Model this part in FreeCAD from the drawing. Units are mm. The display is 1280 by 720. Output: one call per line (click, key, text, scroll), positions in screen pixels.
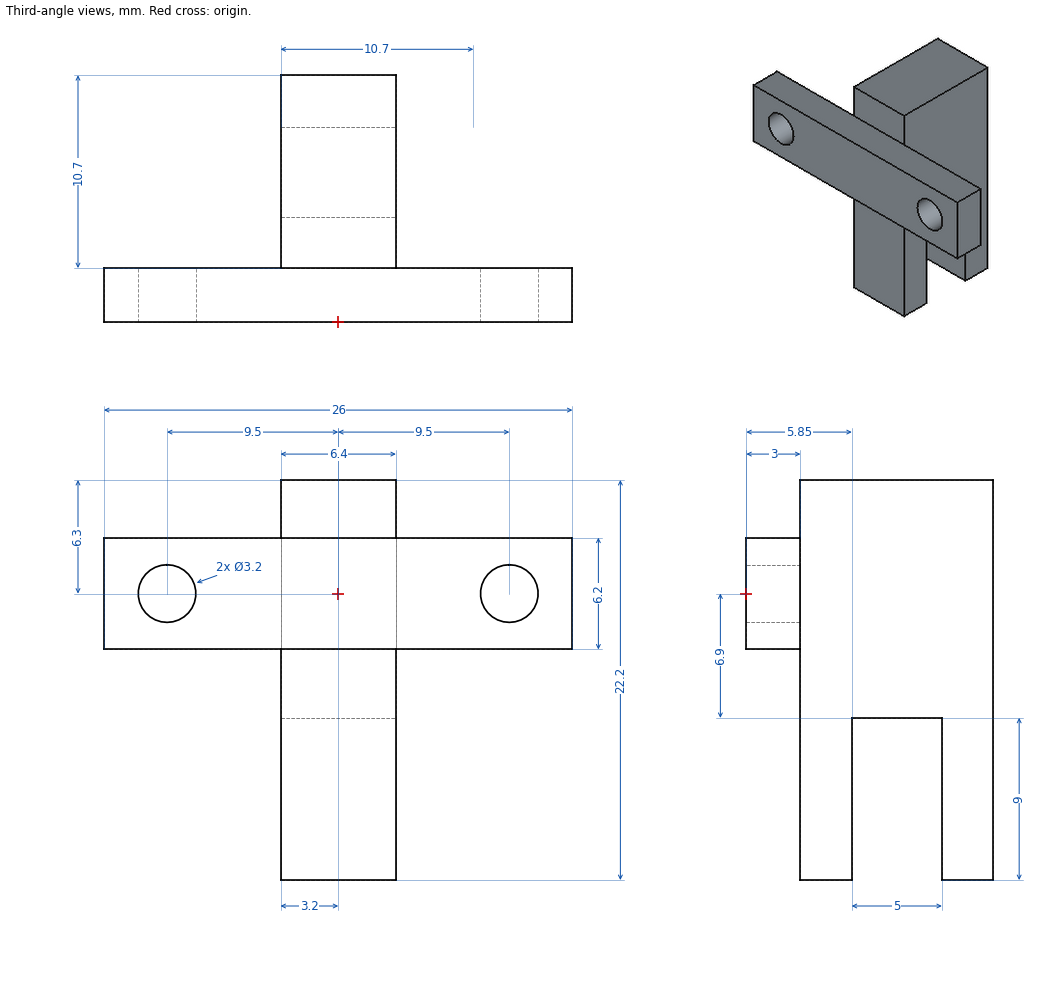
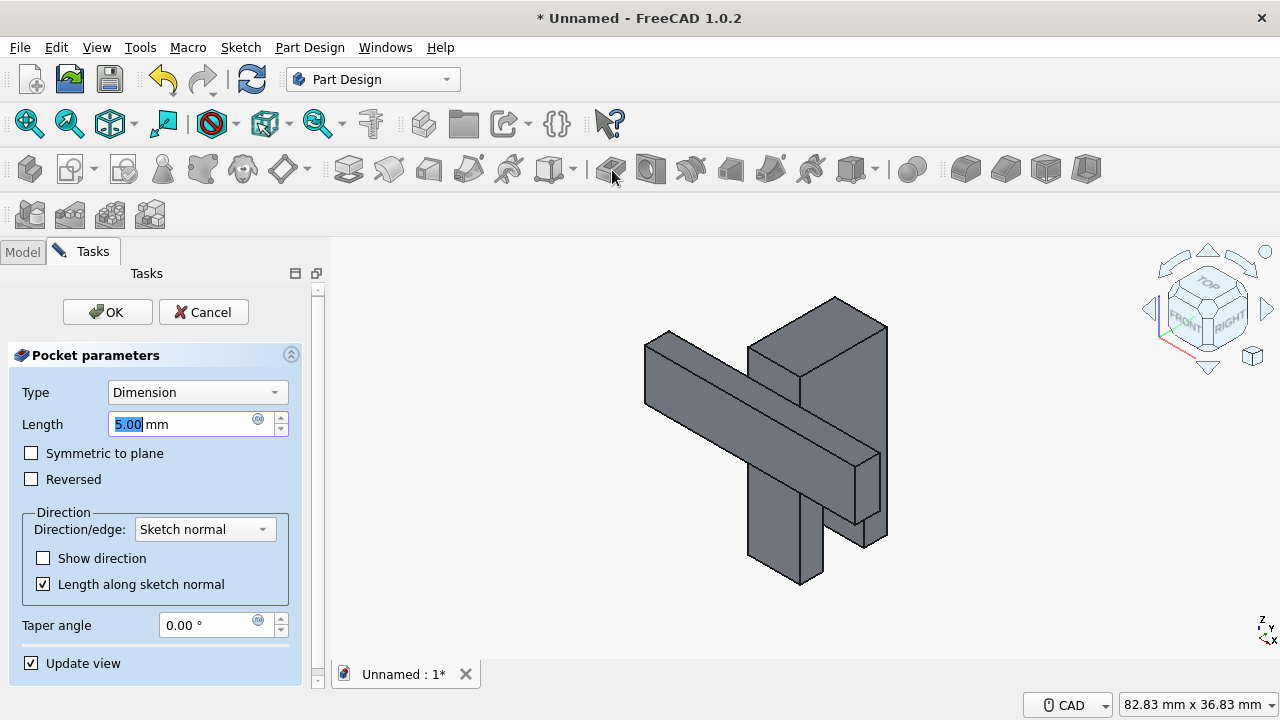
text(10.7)
key(Tab)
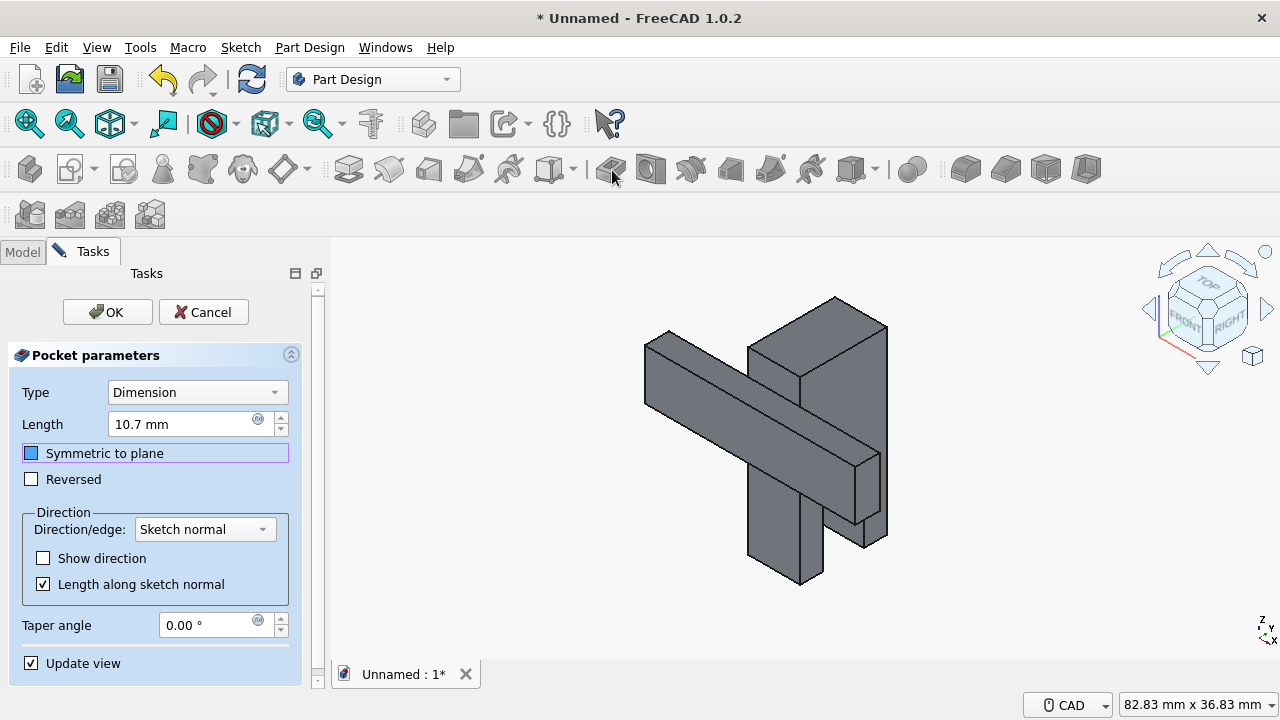
click(30, 479)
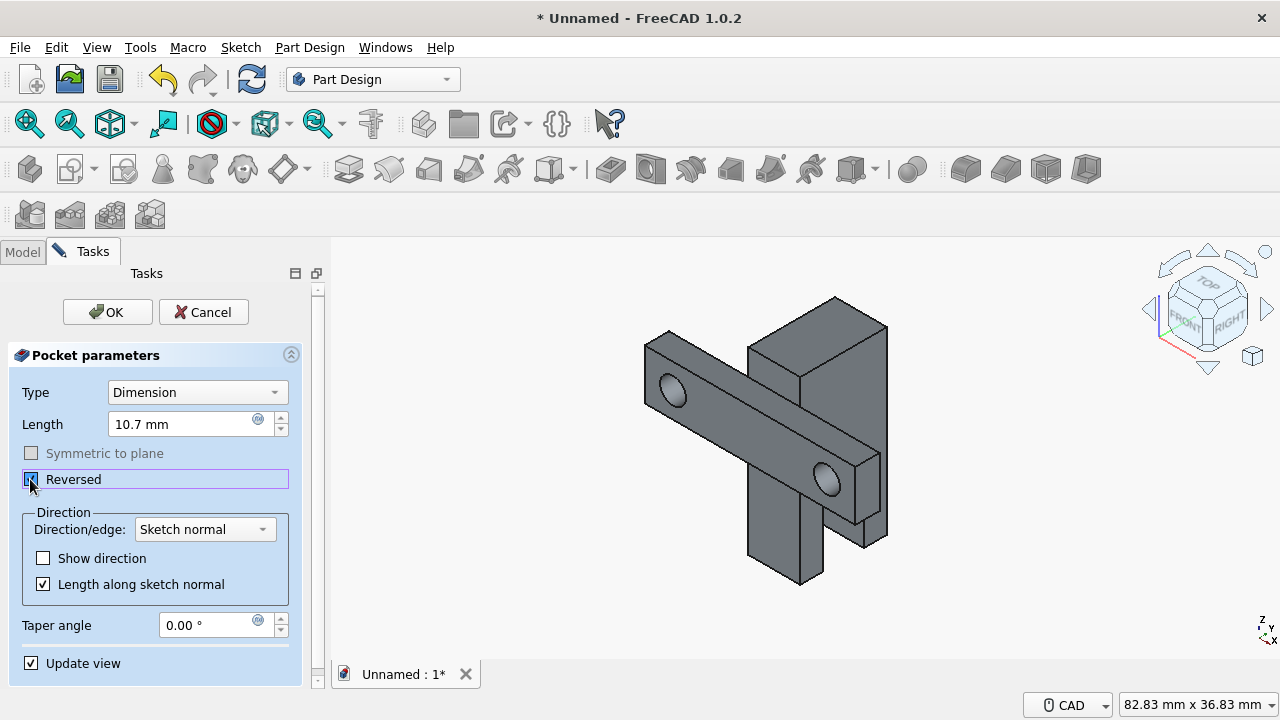
click(108, 312)